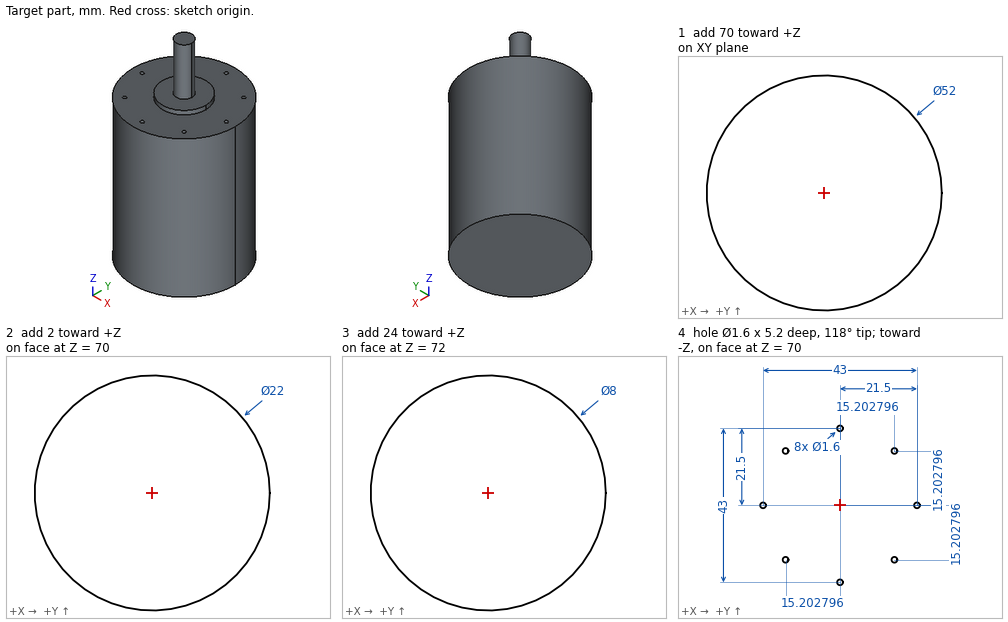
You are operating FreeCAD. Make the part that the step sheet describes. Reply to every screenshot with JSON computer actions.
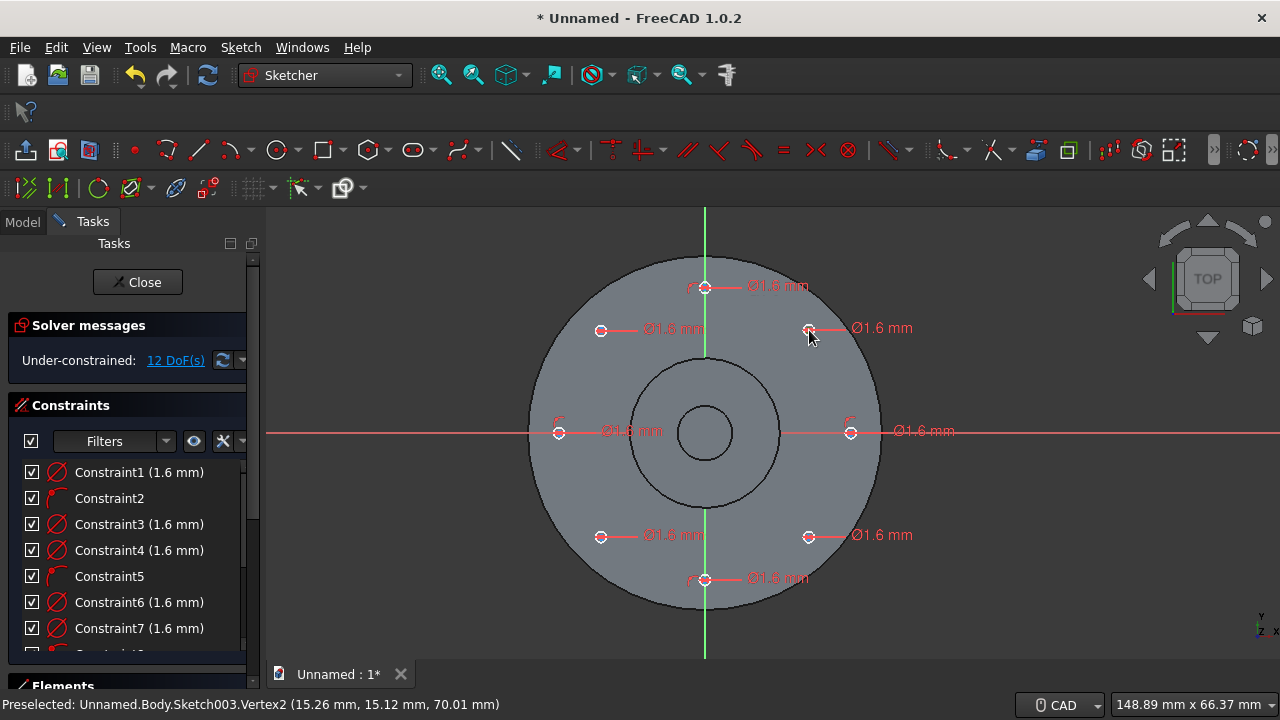
{"action": "left_click", "coordinate": [809, 537]}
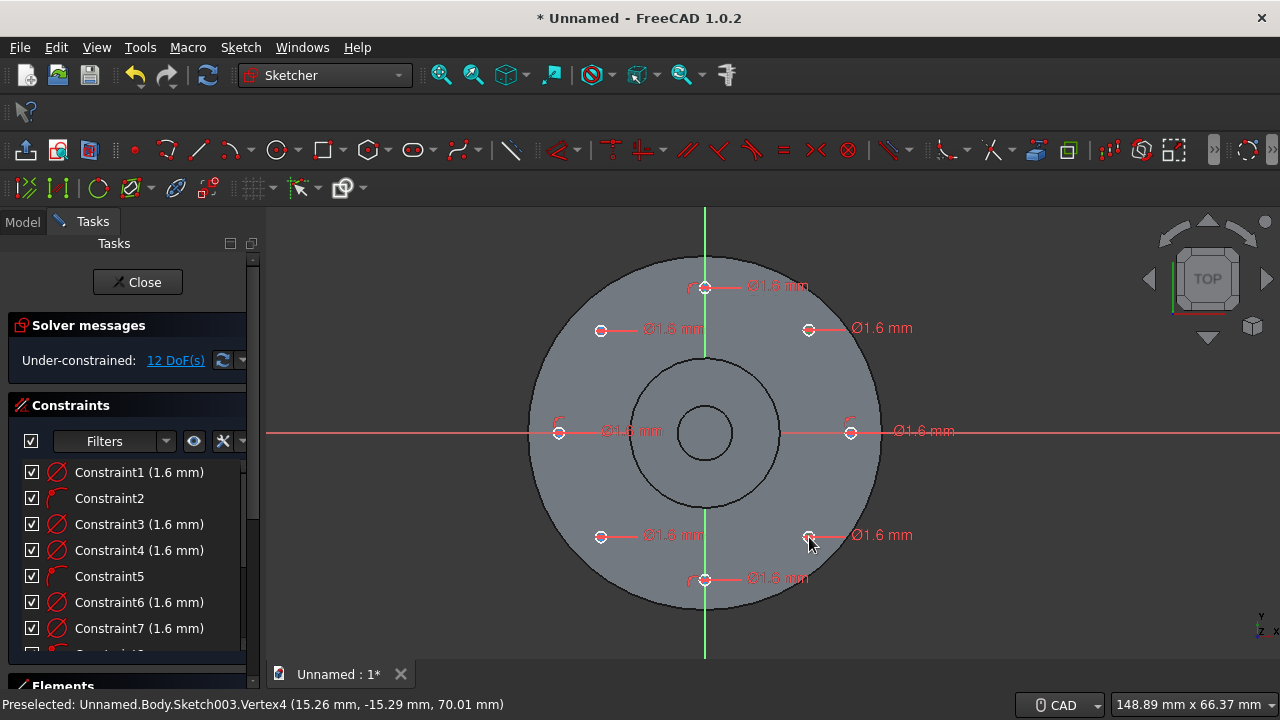
{"action": "key", "text": "v"}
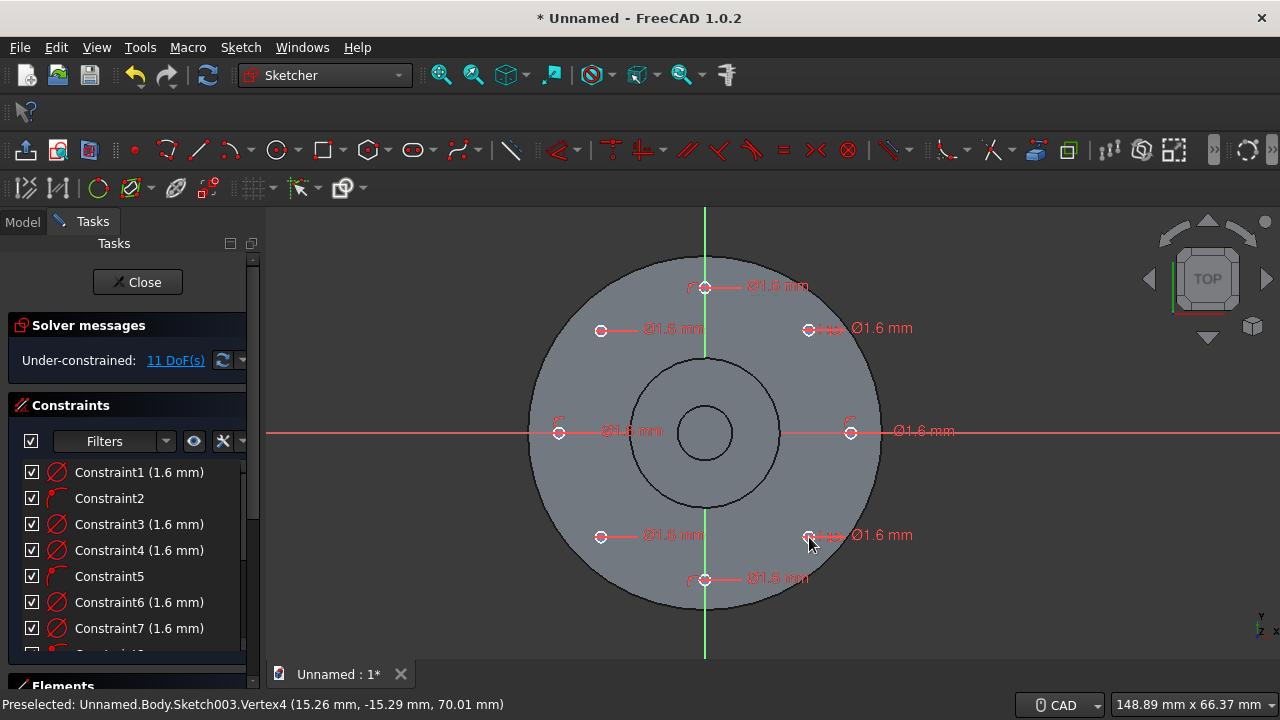
{"action": "left_click", "coordinate": [809, 537]}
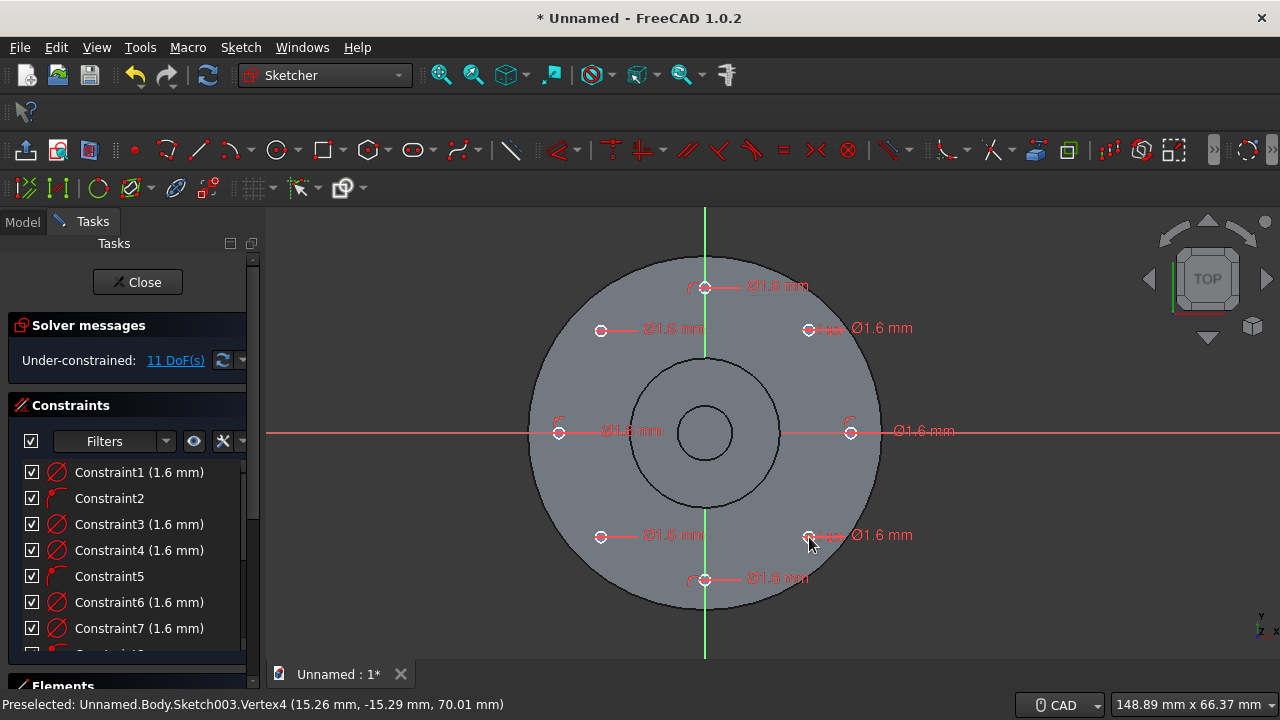
{"action": "left_click", "coordinate": [601, 537]}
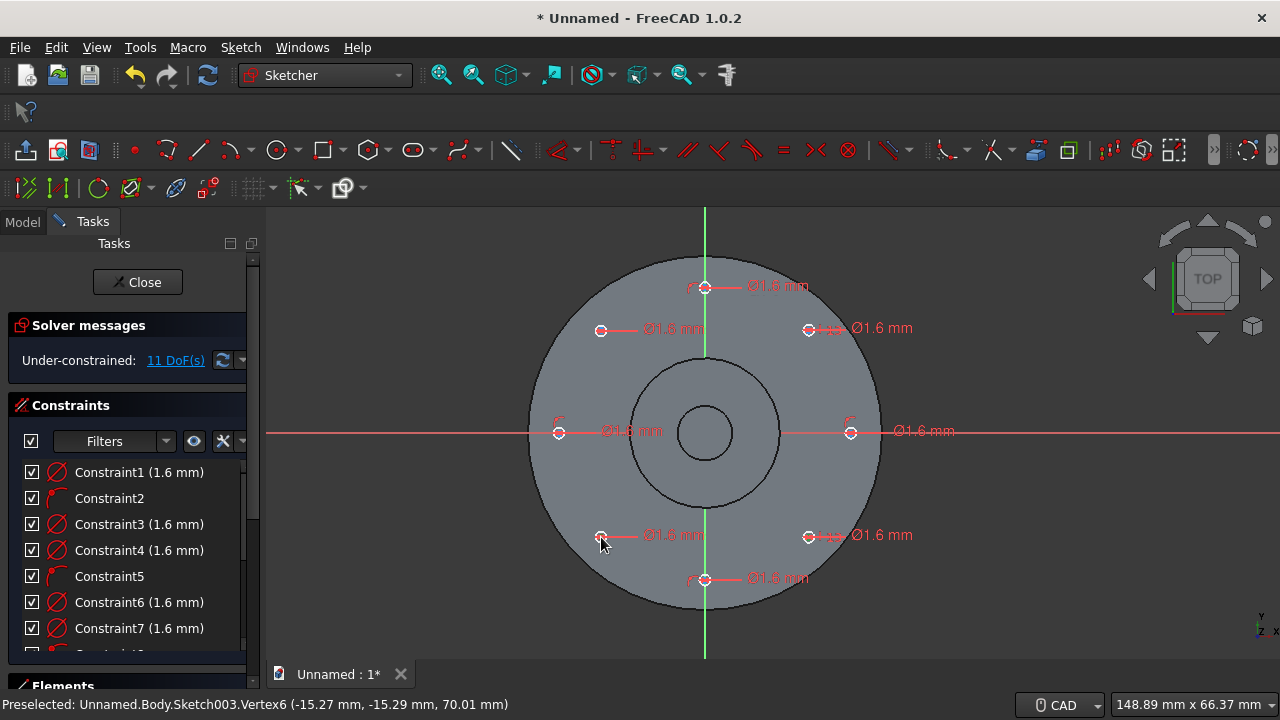
{"action": "key", "text": "h"}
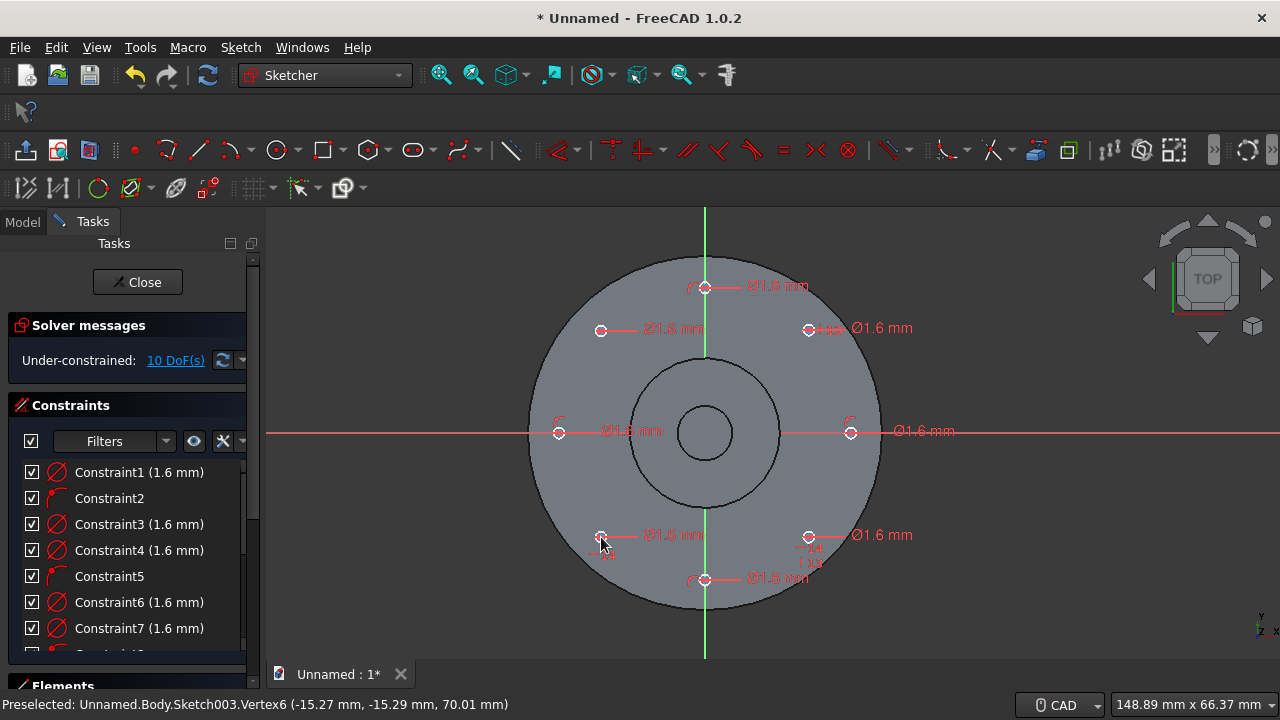
{"action": "left_click", "coordinate": [601, 537]}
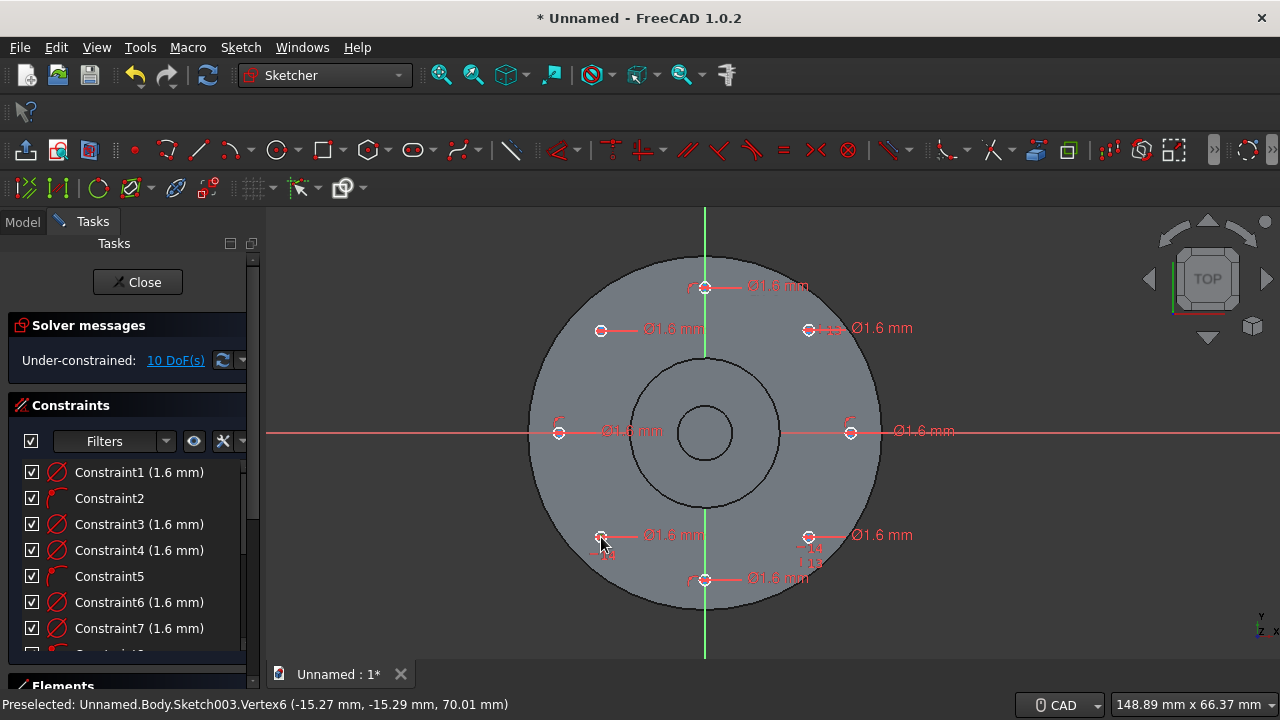
{"action": "left_click", "coordinate": [601, 331]}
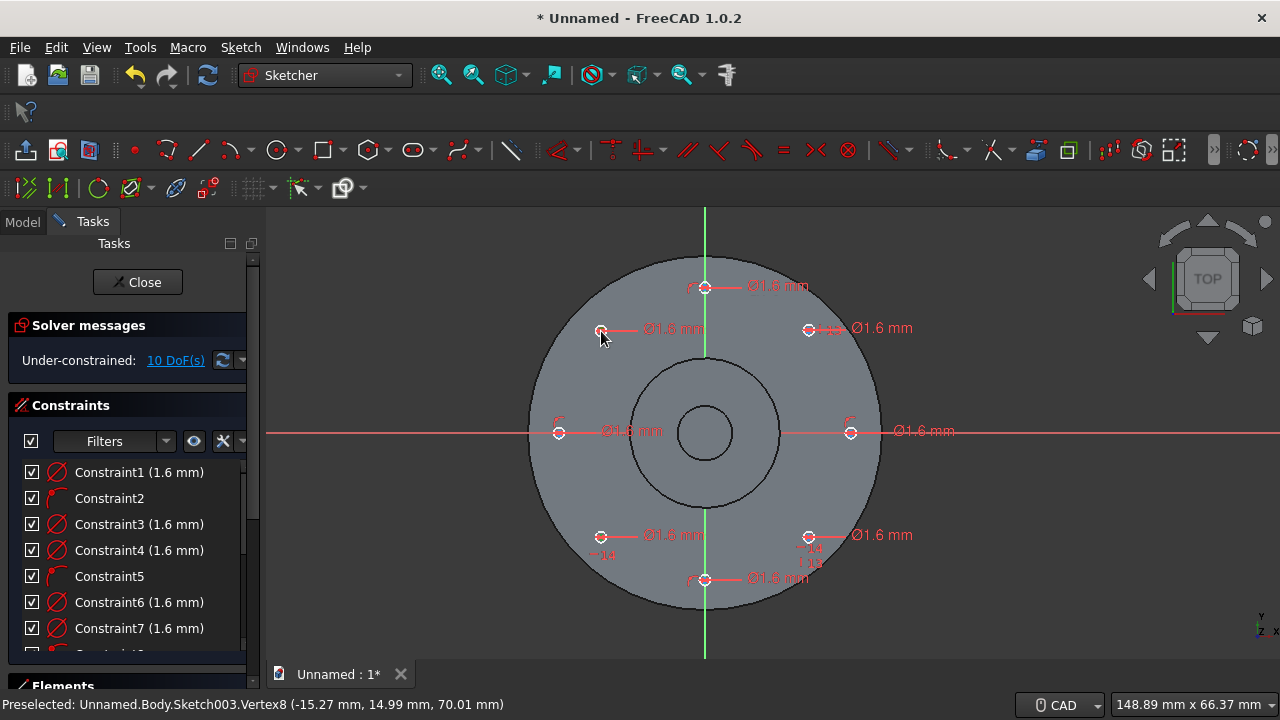
{"action": "left_click", "coordinate": [666, 150]}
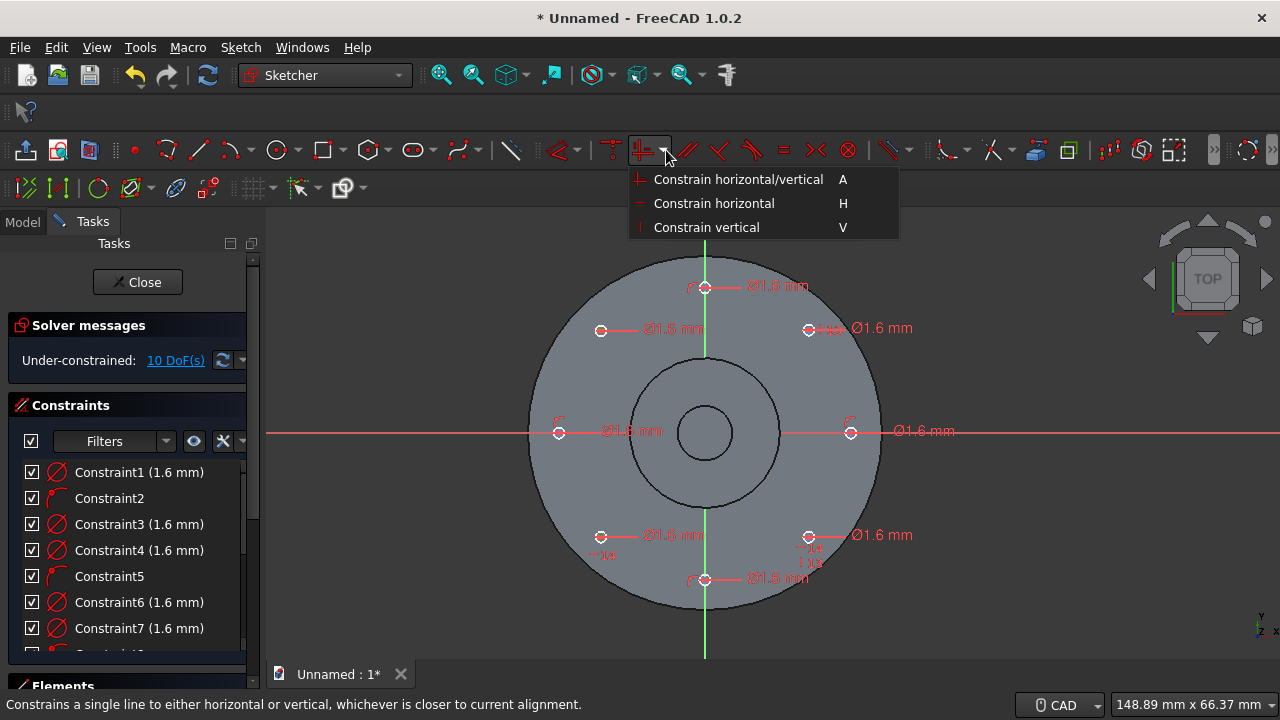
{"action": "left_click", "coordinate": [764, 227]}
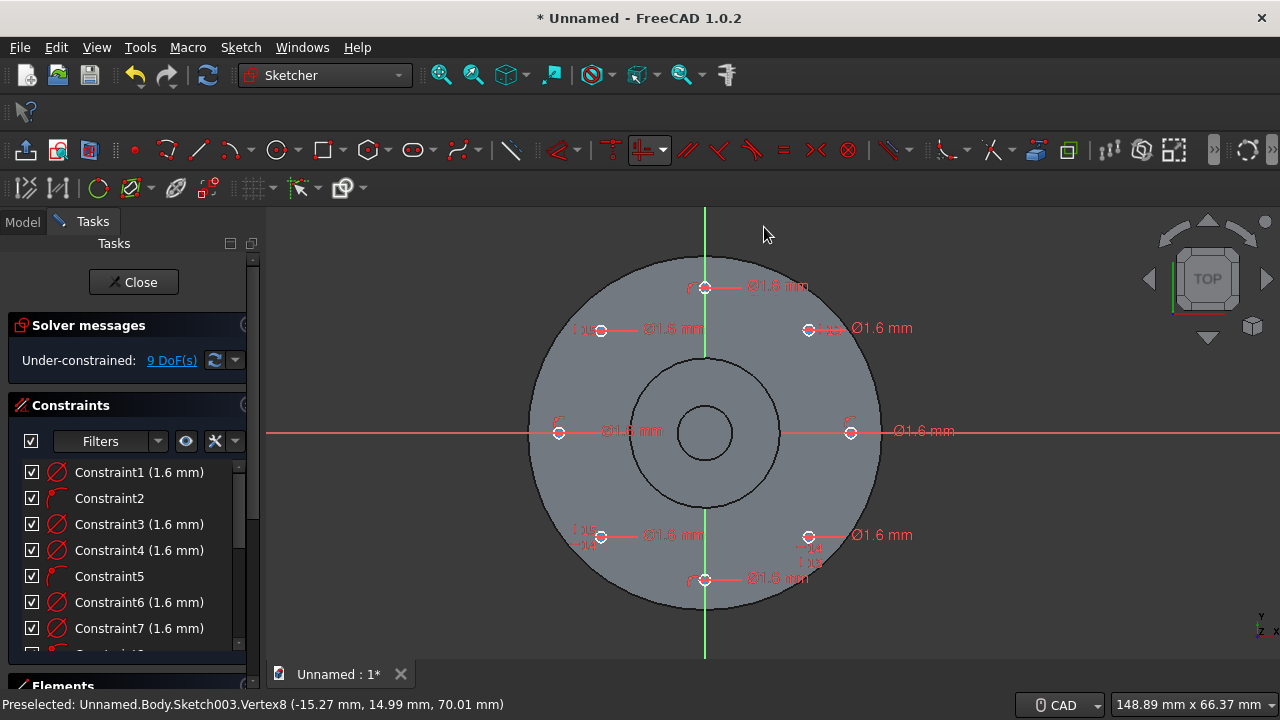
{"action": "left_click", "coordinate": [809, 330]}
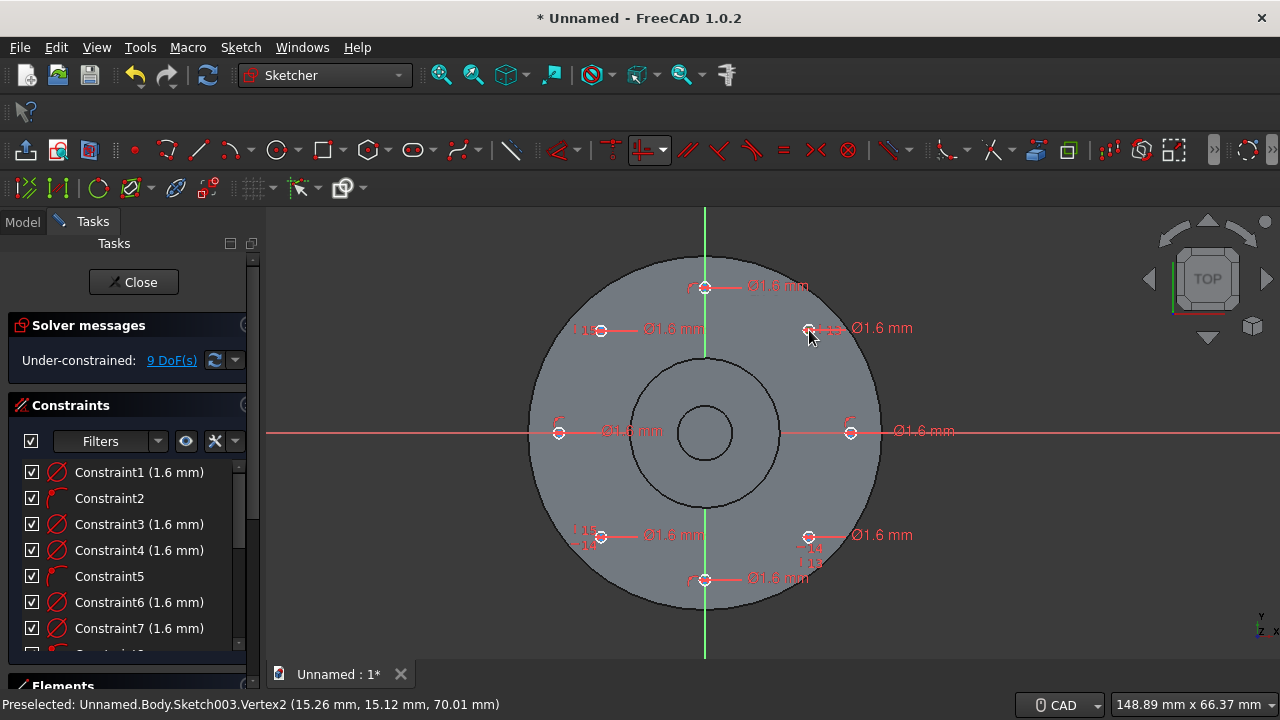
{"action": "left_click", "coordinate": [601, 331]}